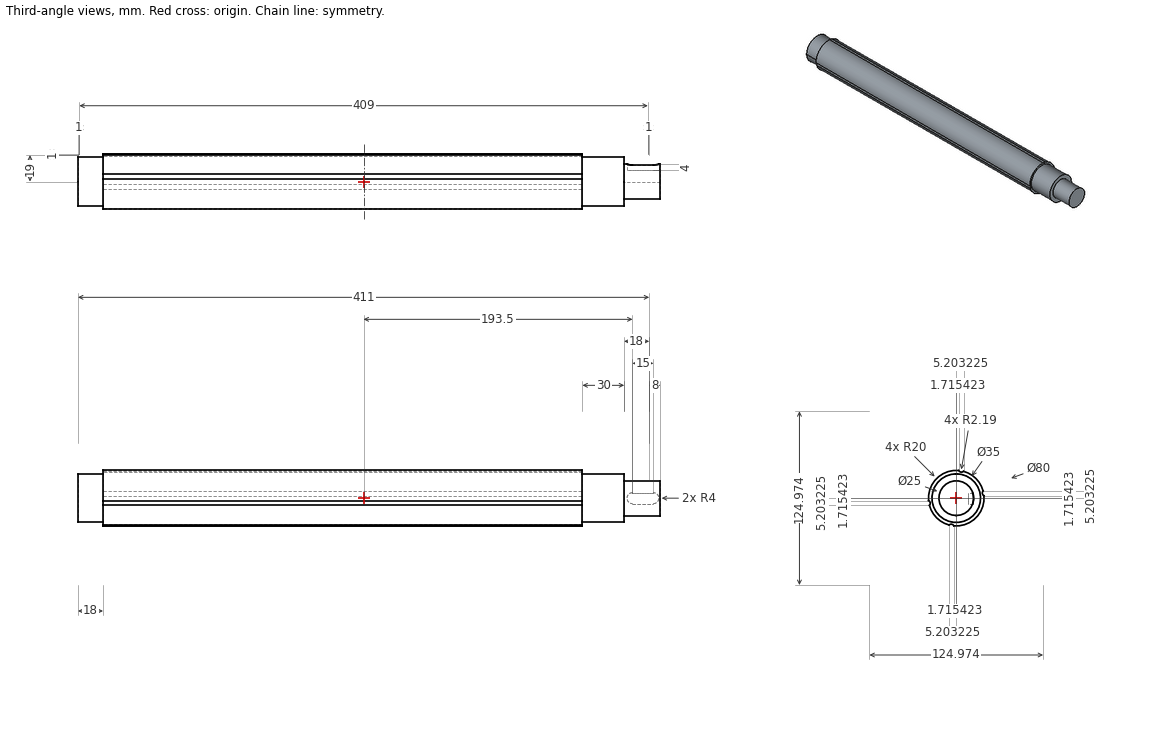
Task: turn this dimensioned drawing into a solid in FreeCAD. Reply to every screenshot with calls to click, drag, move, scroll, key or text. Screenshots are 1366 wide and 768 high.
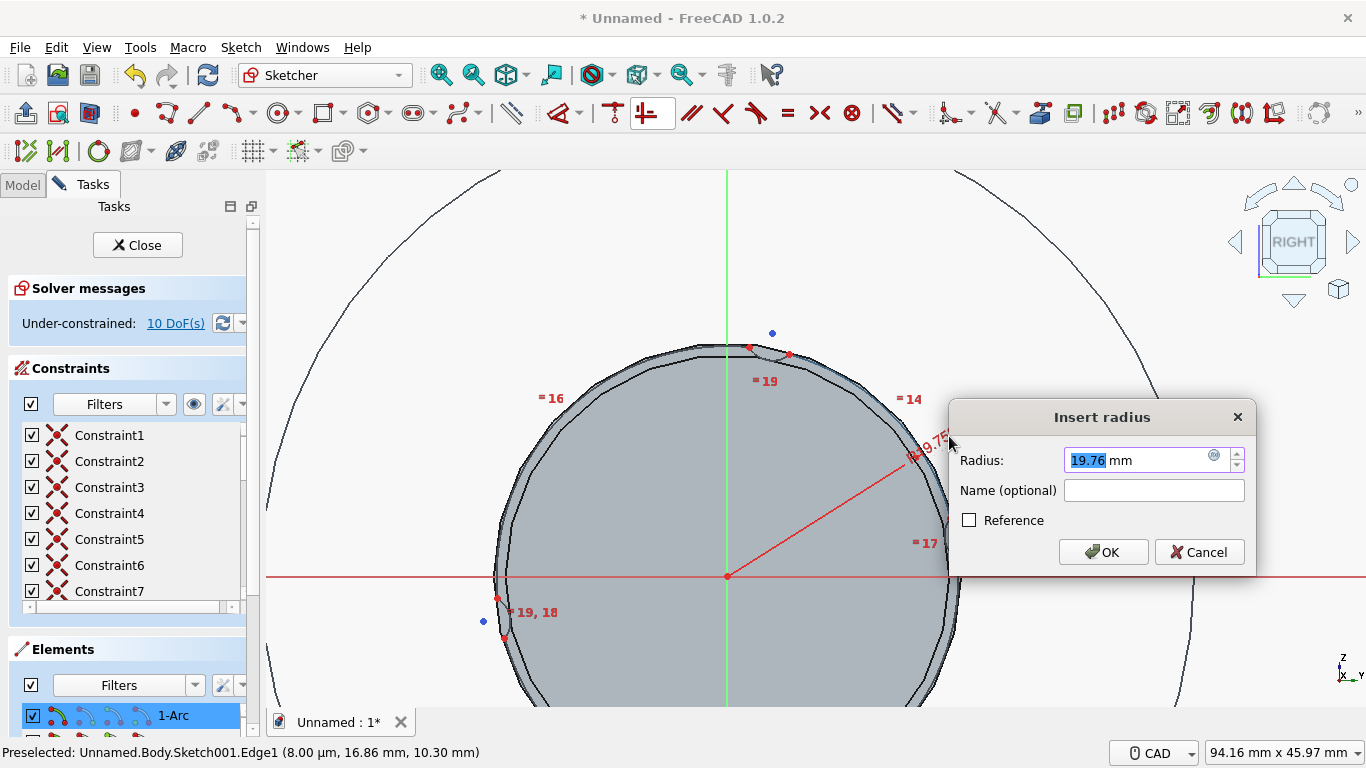
text(20)
key(Return)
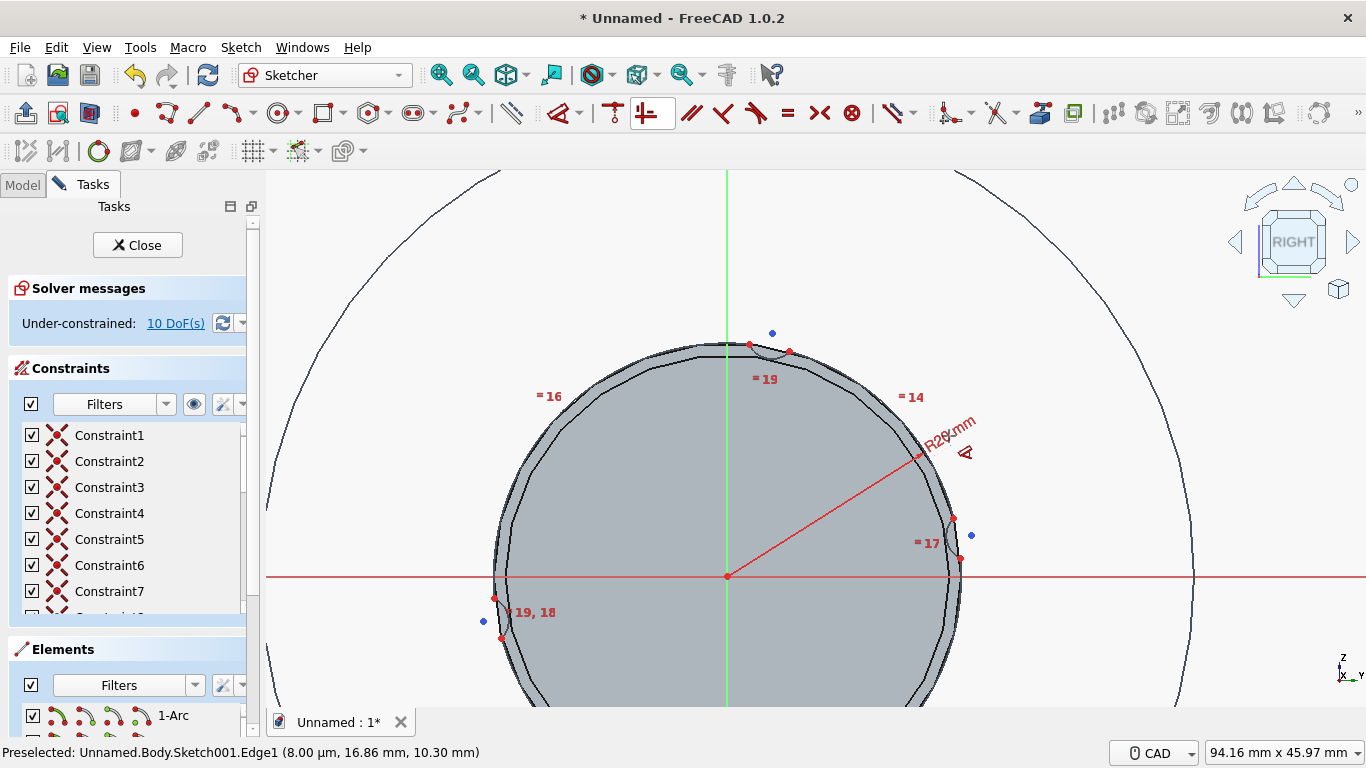
scroll(947, 531, up, 3)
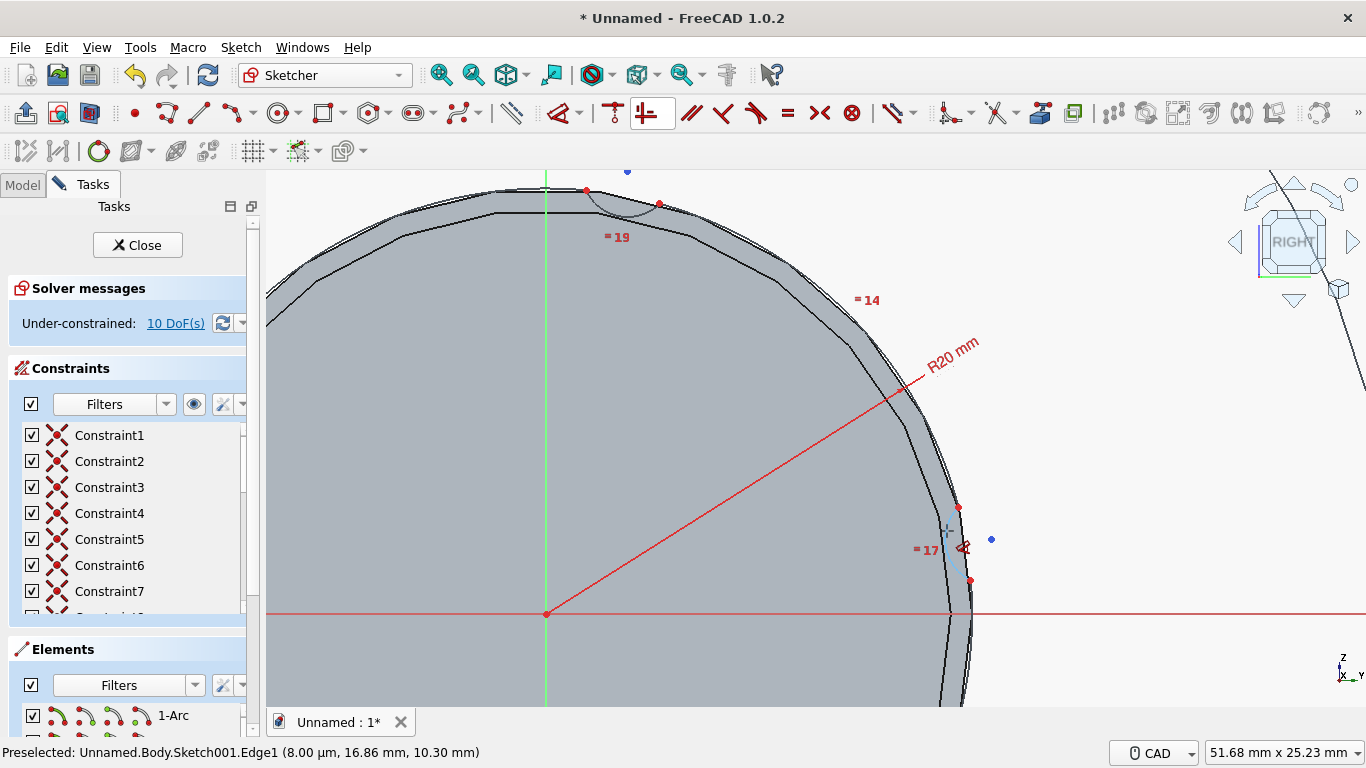
click(946, 530)
click(915, 523)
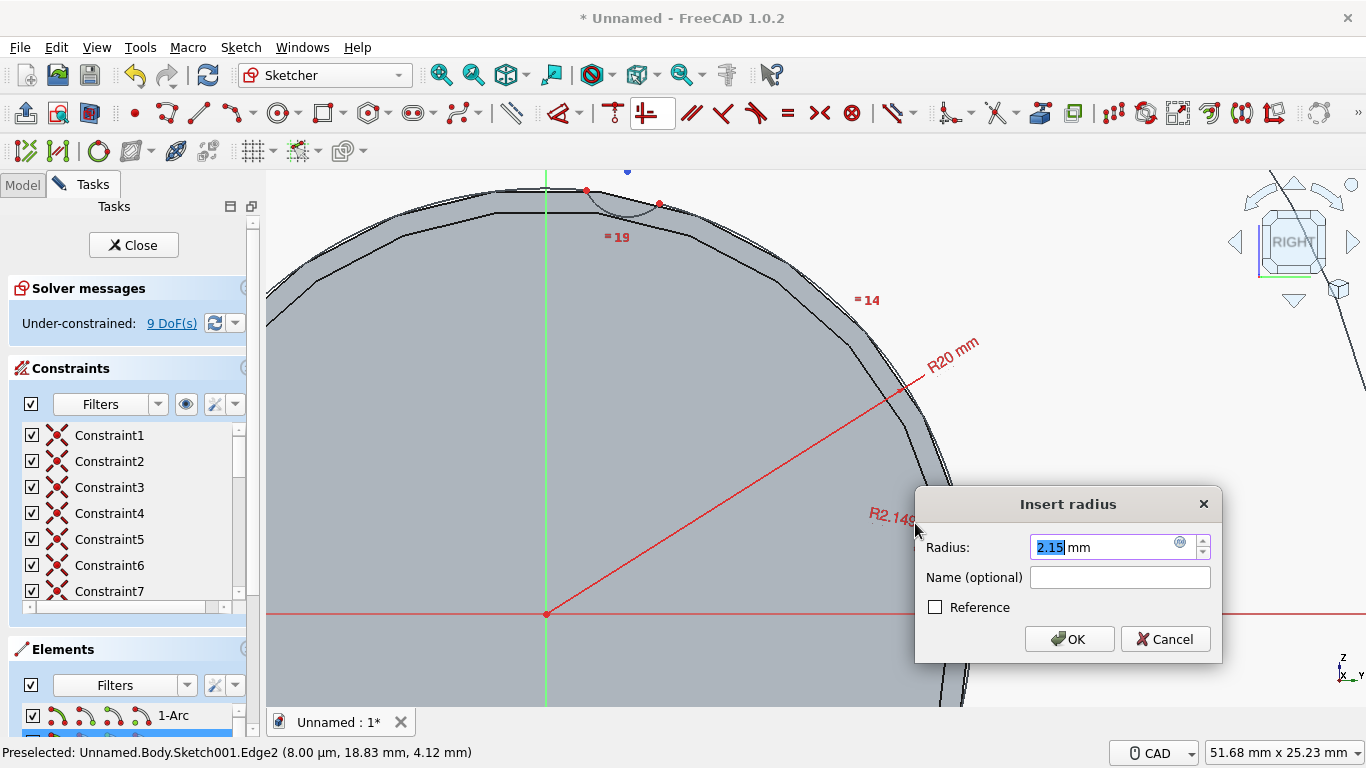
text(2.19)
key(Return)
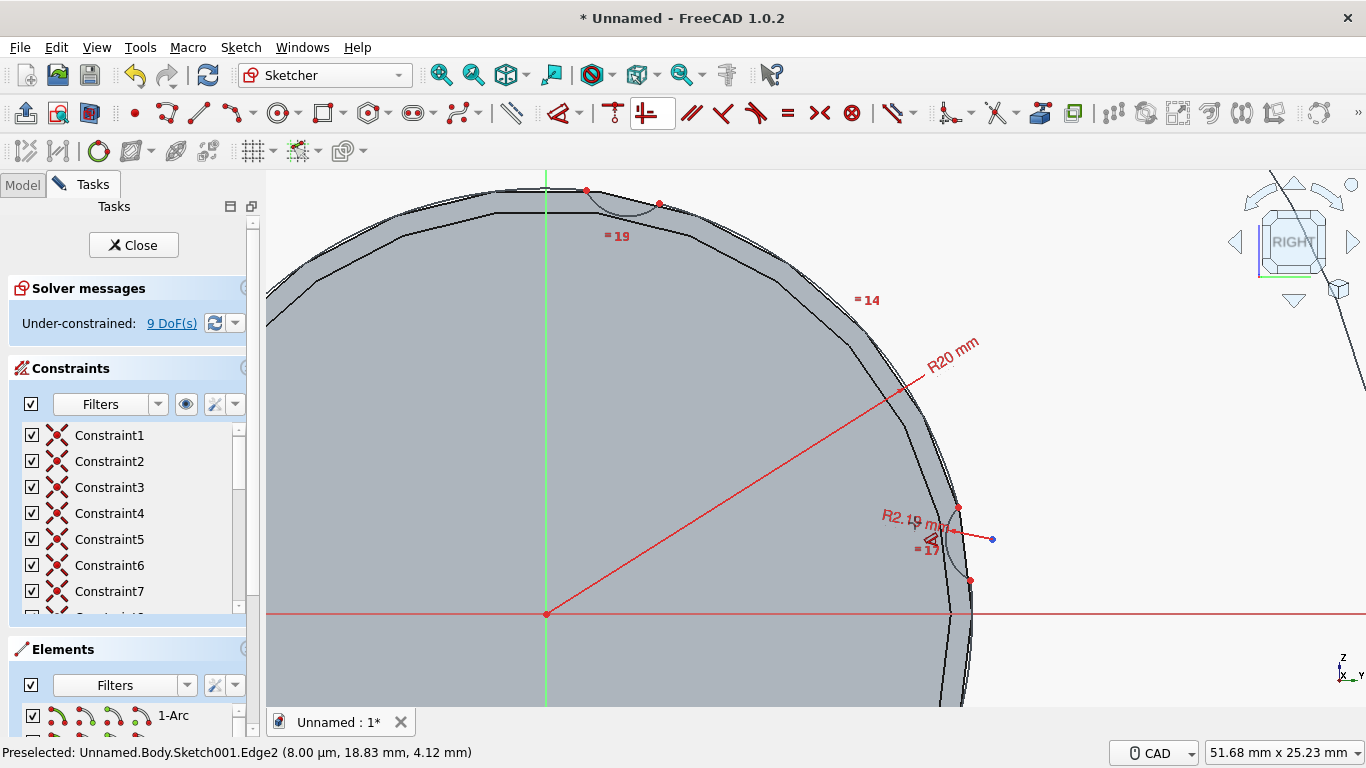
scroll(798, 394, down, 8)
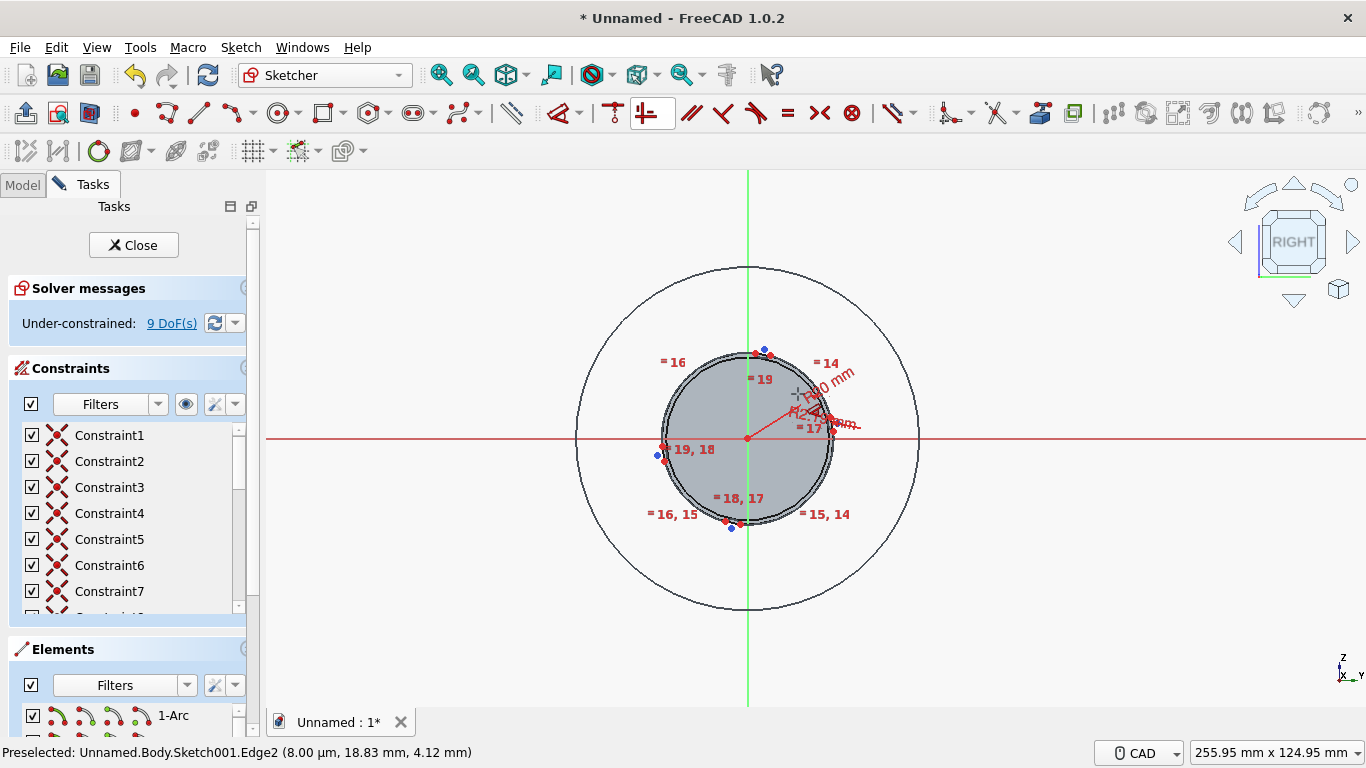
click(869, 317)
click(892, 294)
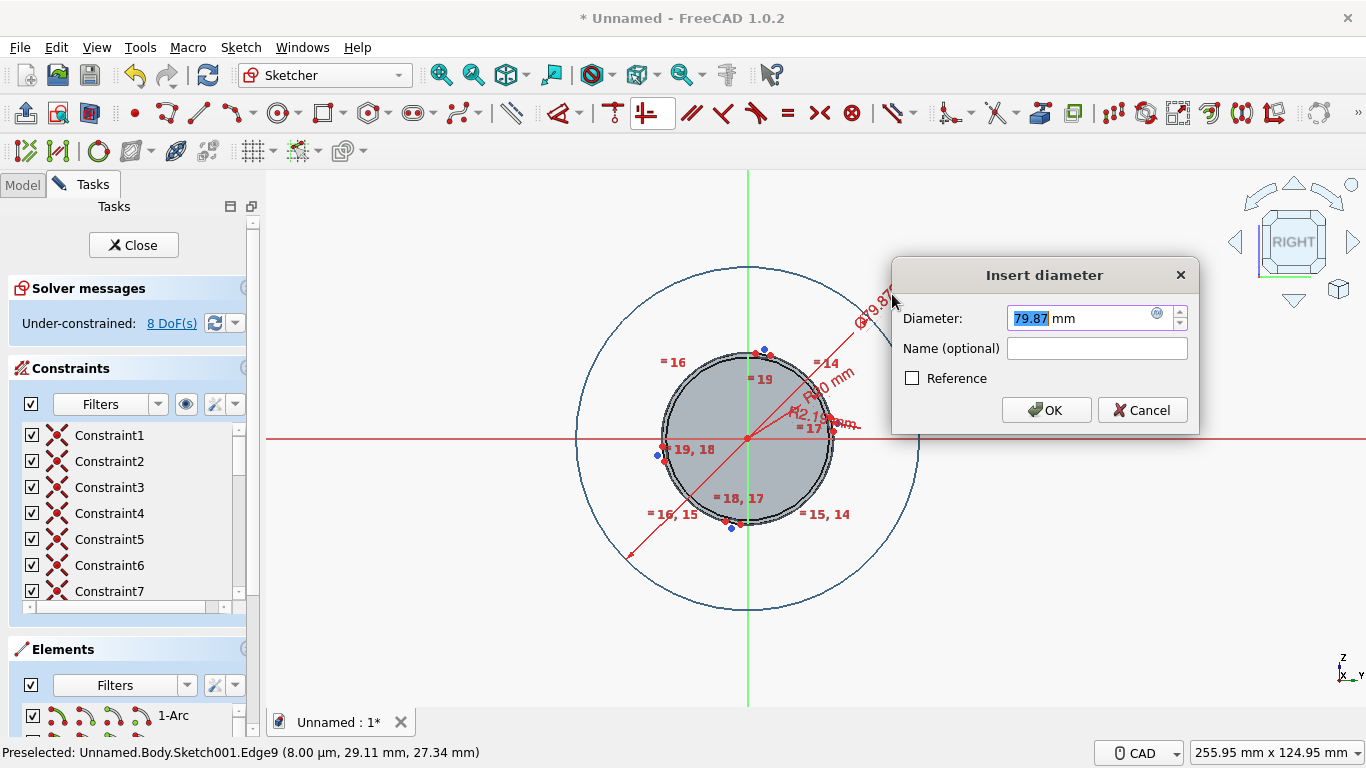
text(80)
key(Return)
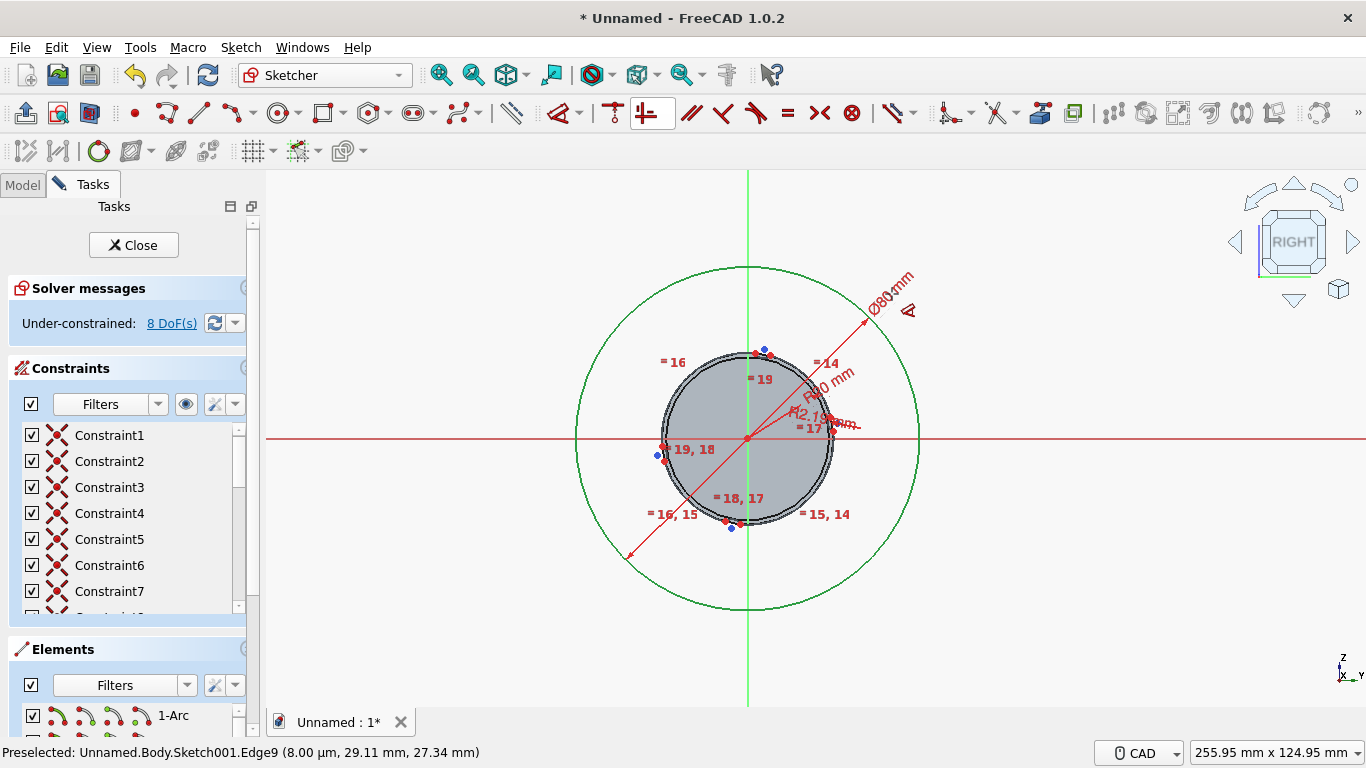
scroll(831, 417, up, 3)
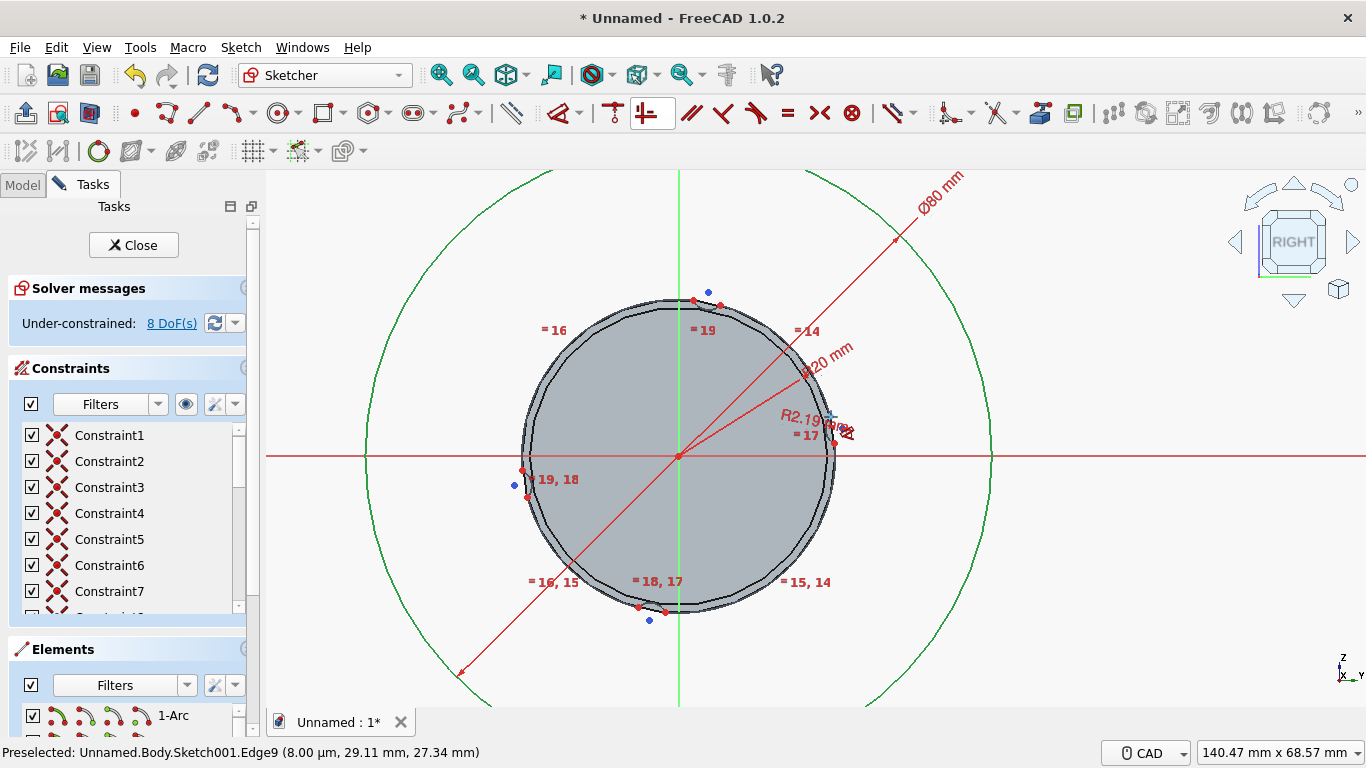
click(830, 417)
click(645, 437)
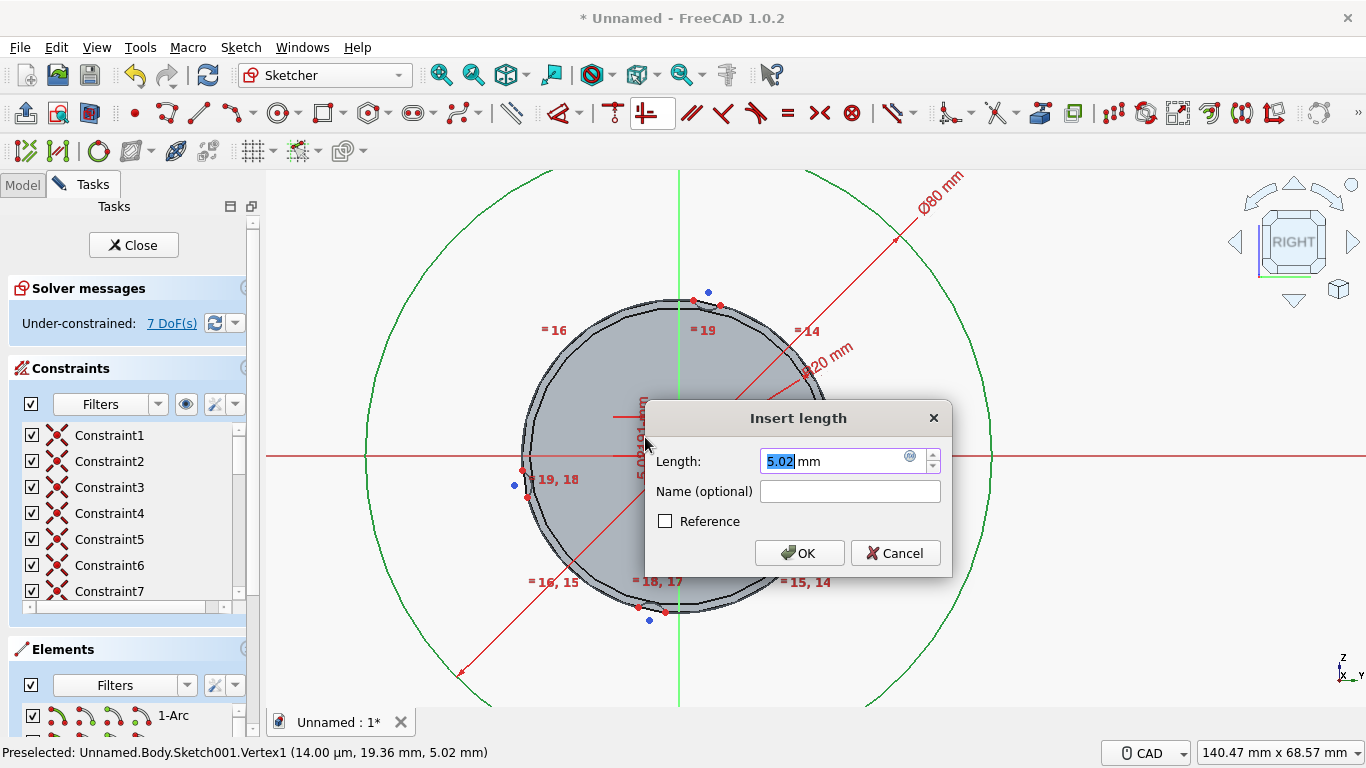
text(5.203225)
key(Return)